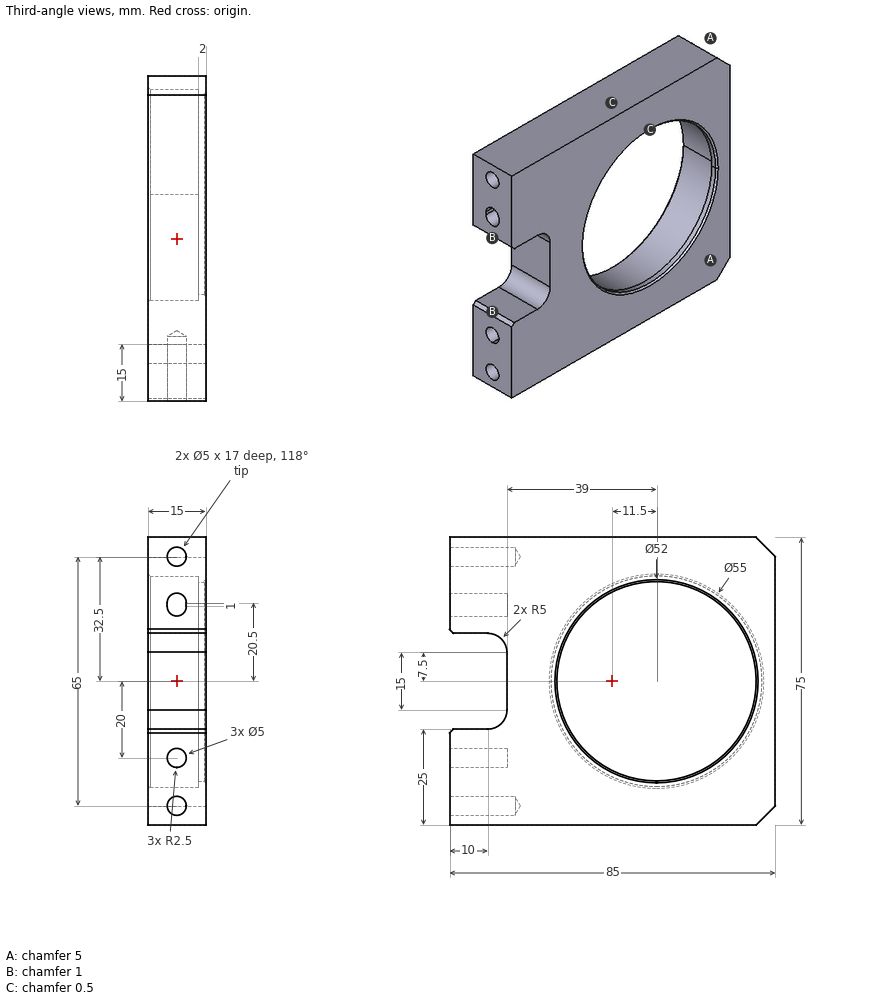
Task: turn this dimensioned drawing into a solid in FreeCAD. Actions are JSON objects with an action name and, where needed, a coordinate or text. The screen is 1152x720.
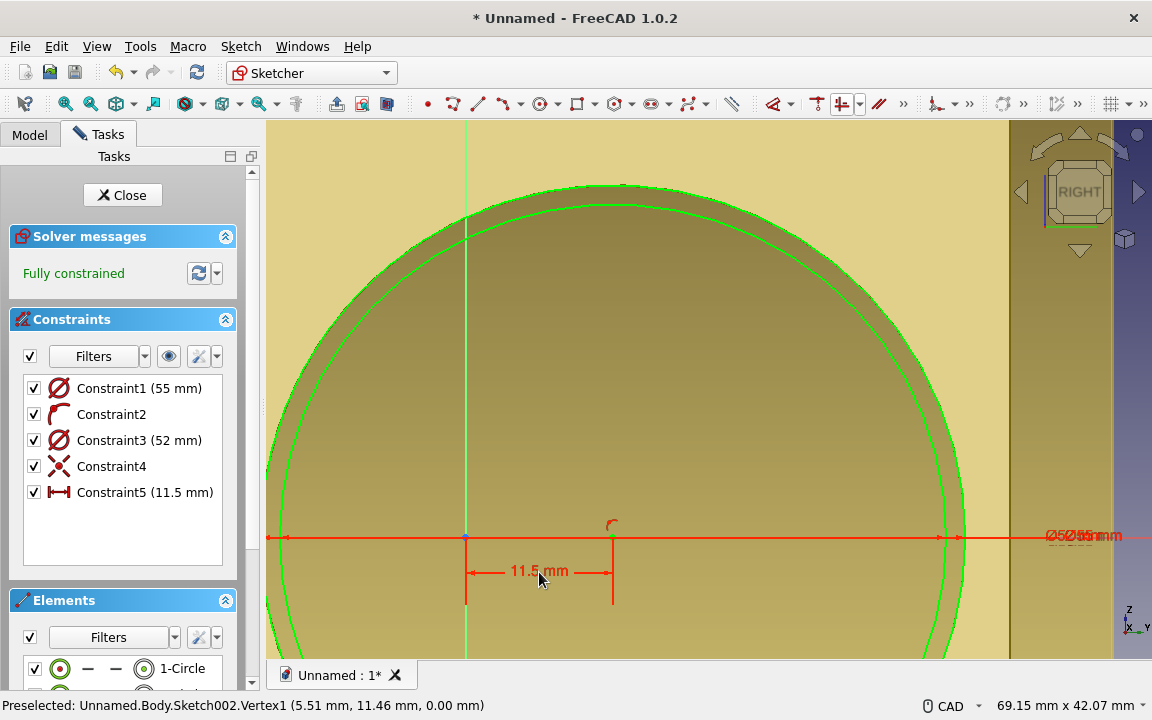
{"action": "left_click", "coordinate": [123, 195]}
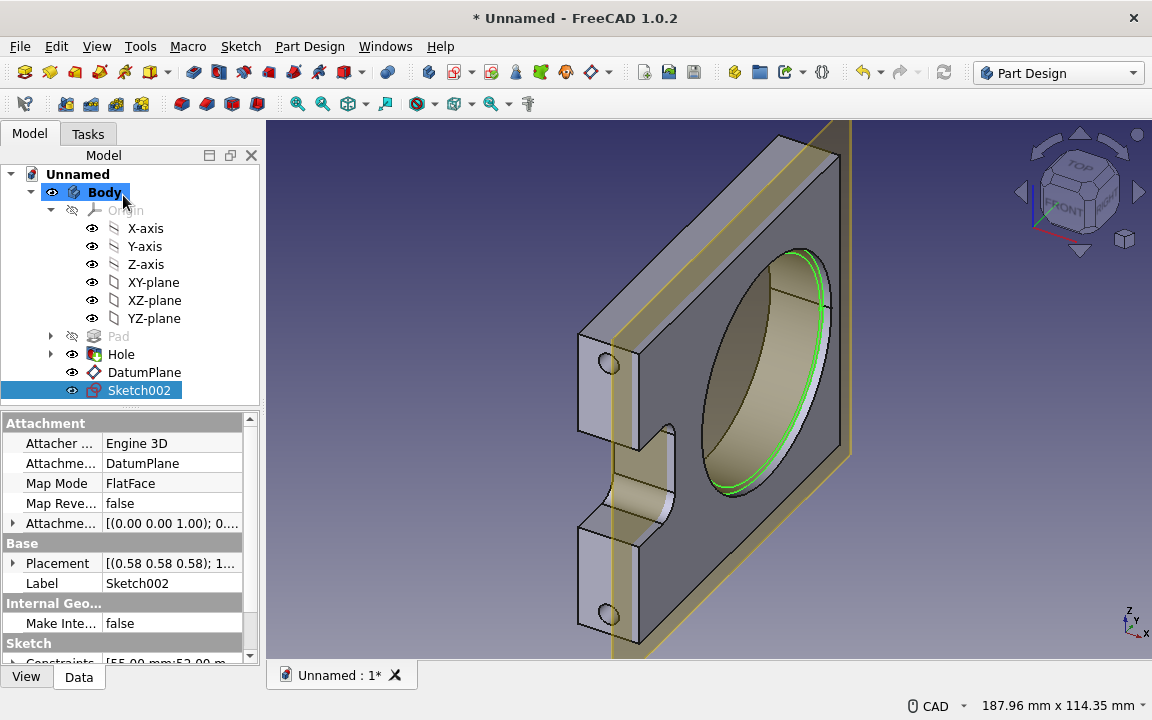
{"action": "left_click", "coordinate": [25, 72]}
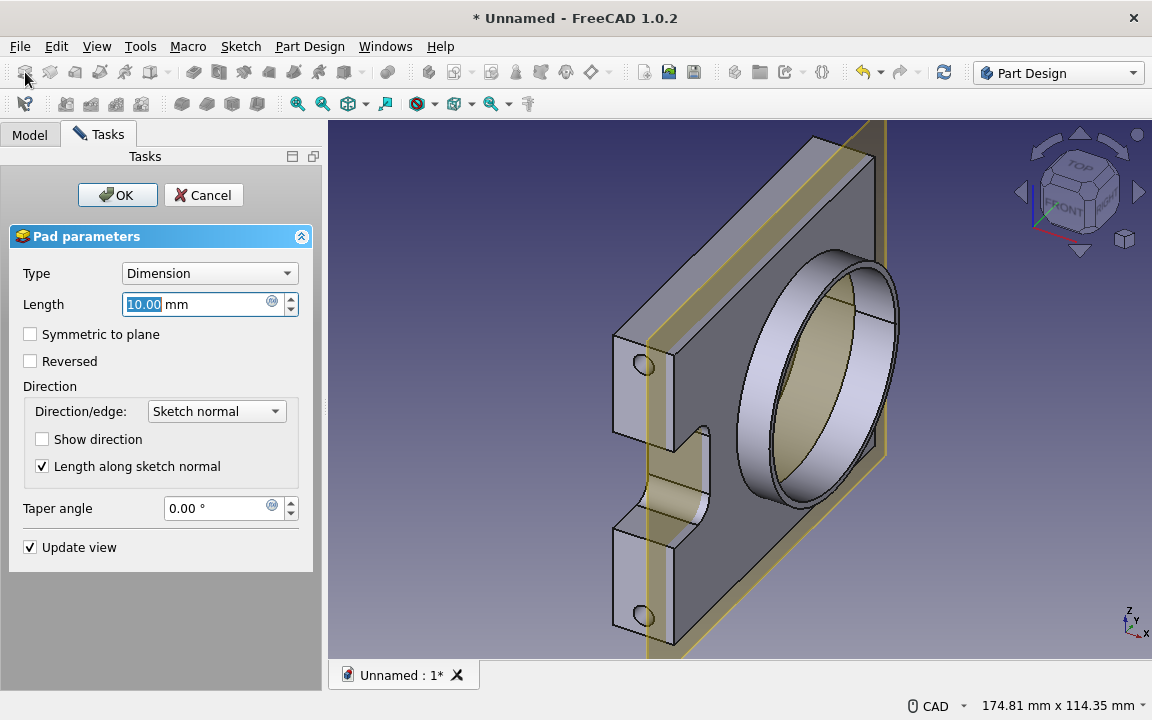
{"action": "type", "text": "2"}
{"action": "key", "text": "Tab"}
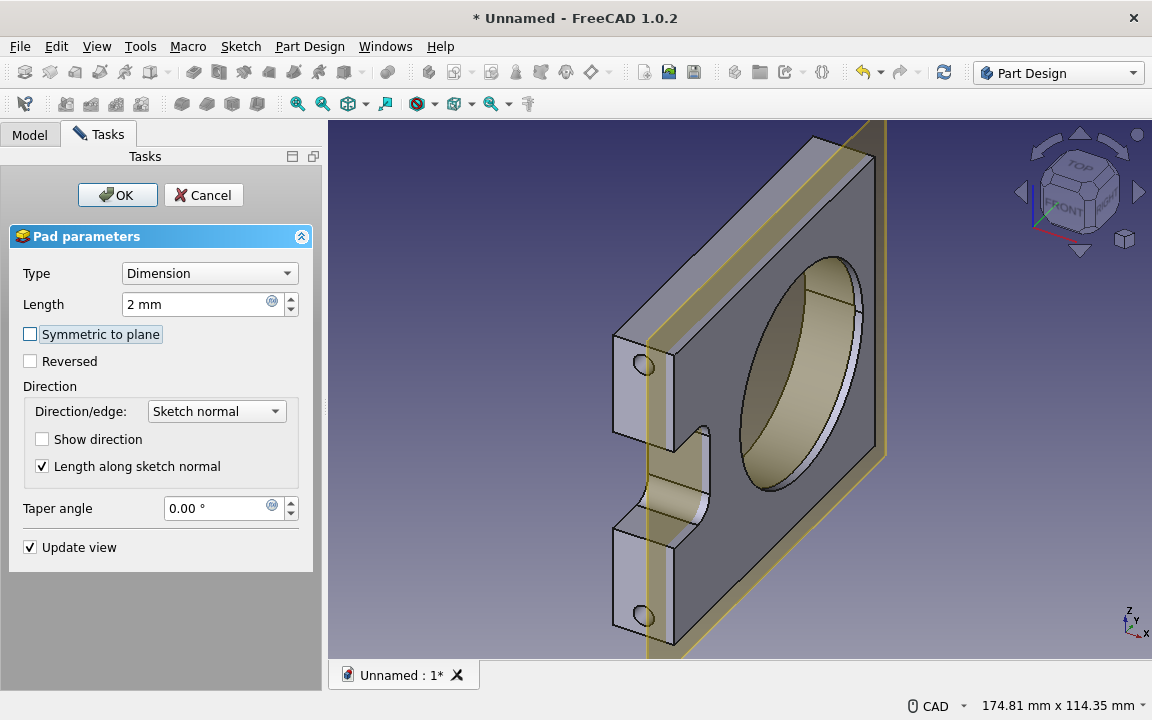
{"action": "left_click", "coordinate": [118, 195]}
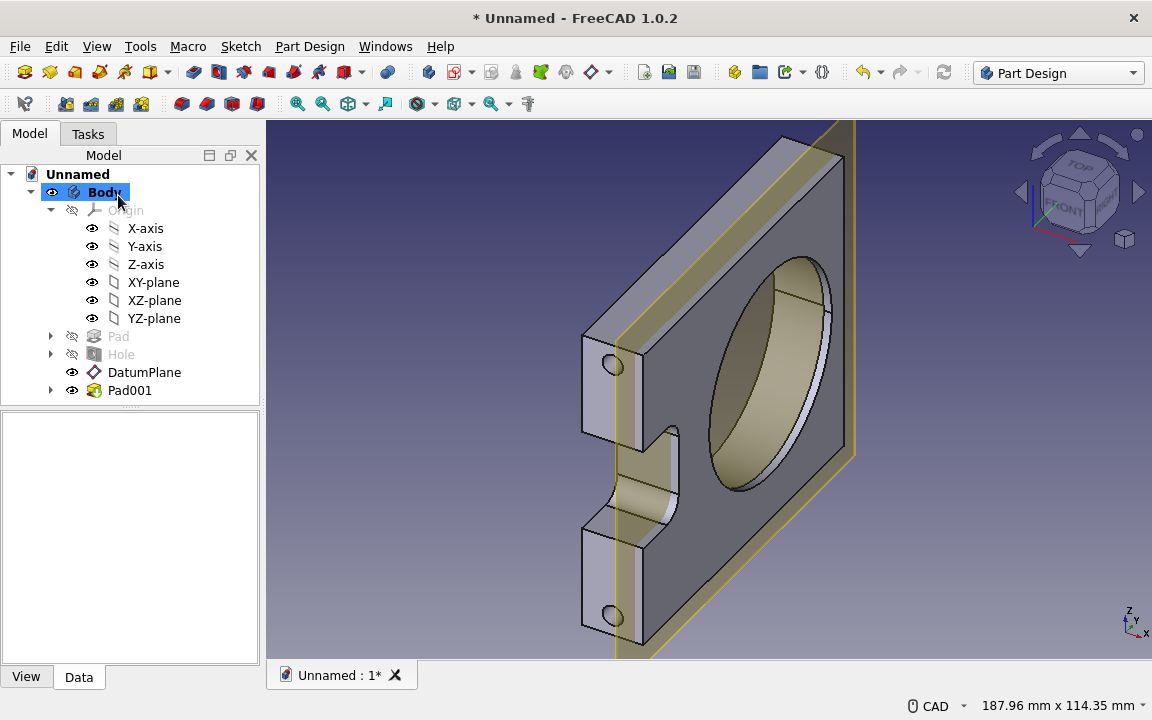
{"action": "left_click", "coordinate": [117, 372]}
{"action": "key", "text": "space"}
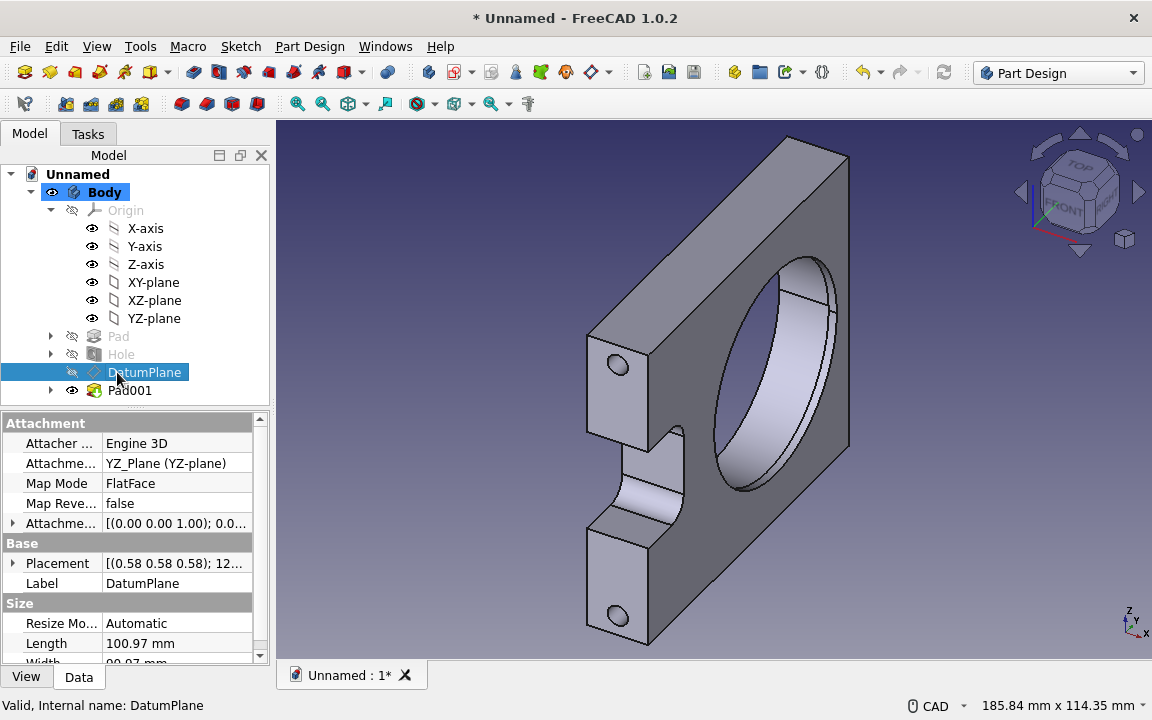
{"action": "key", "text": "0"}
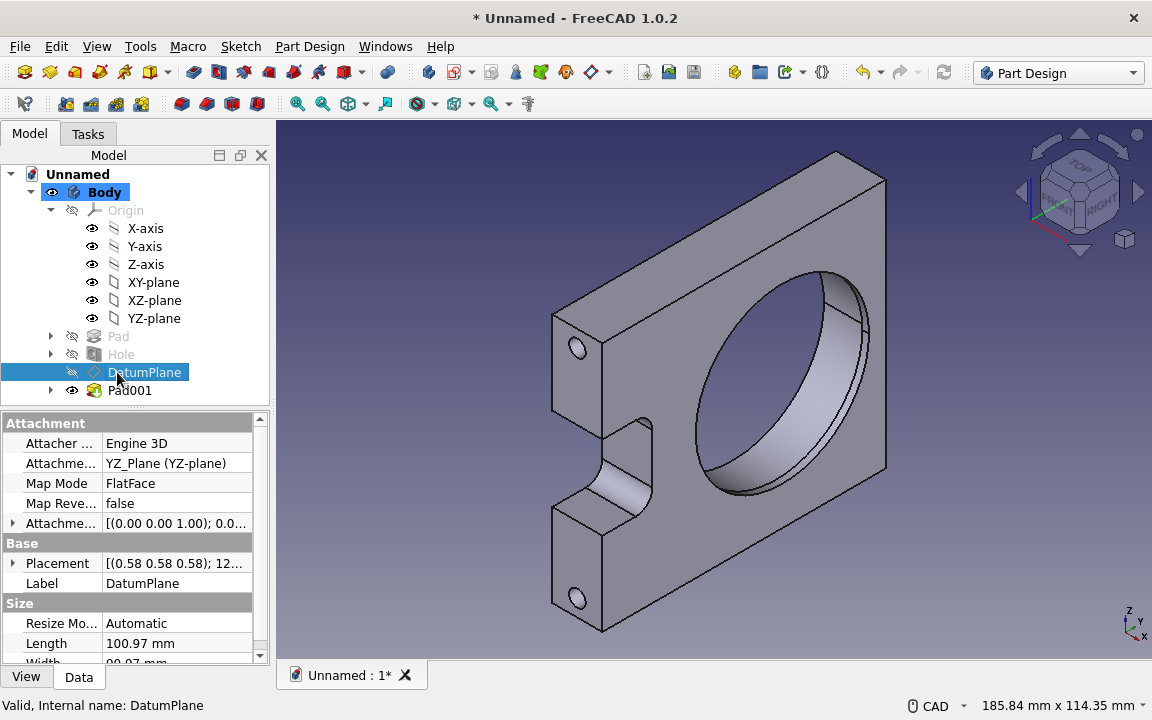
{"action": "key", "text": "2"}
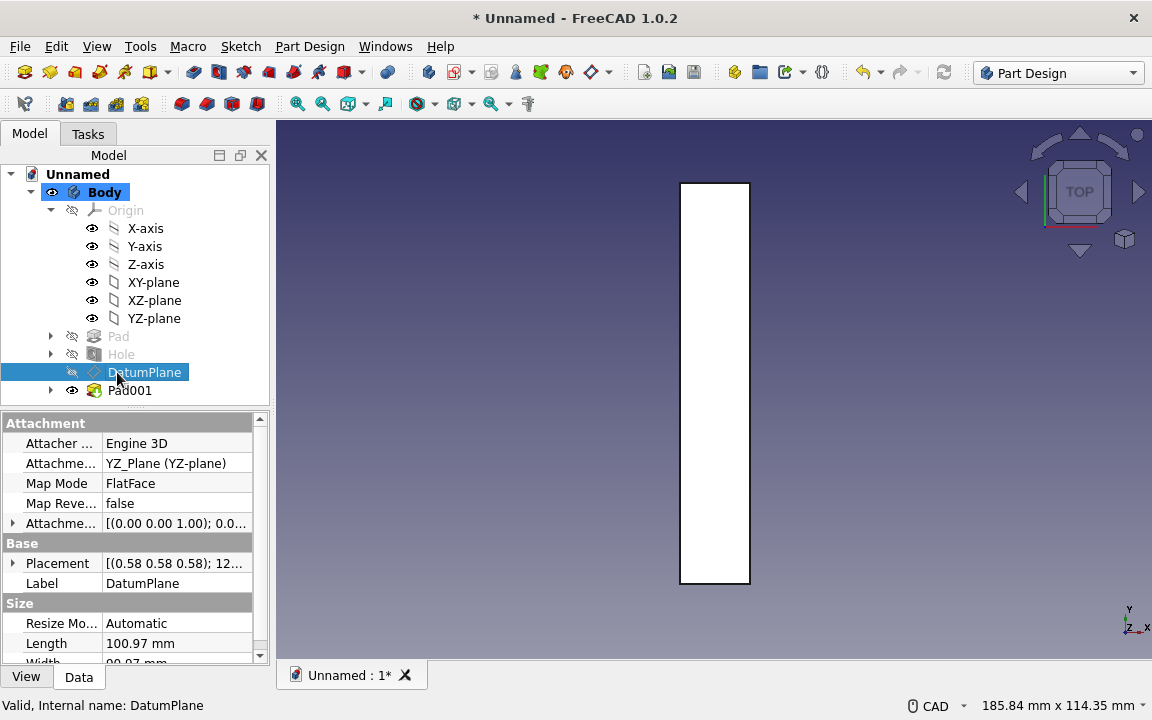
{"action": "left_click", "coordinate": [715, 182]}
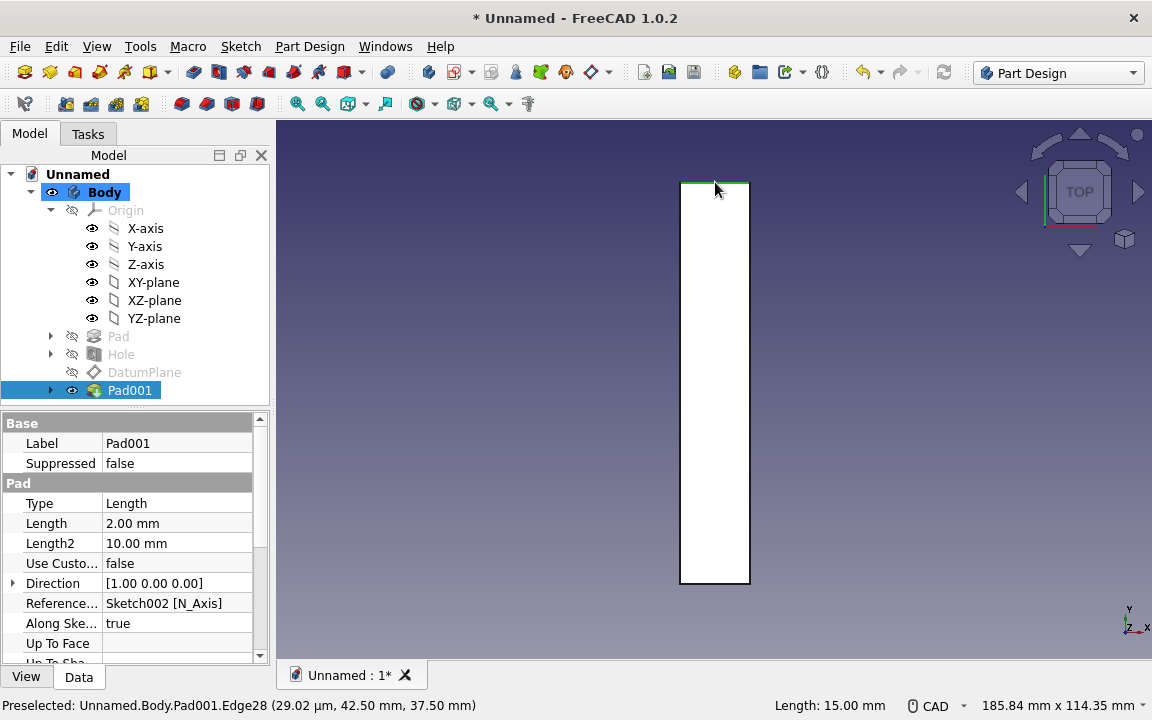
{"action": "key", "text": "1"}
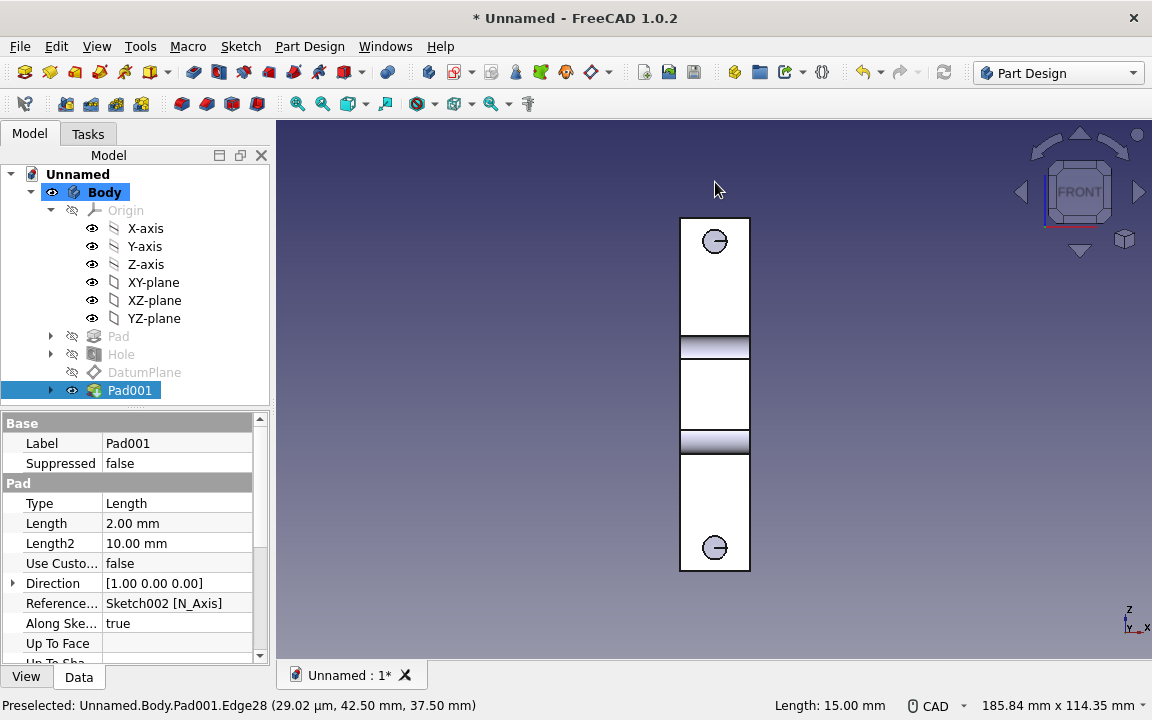
{"action": "key", "text": "3"}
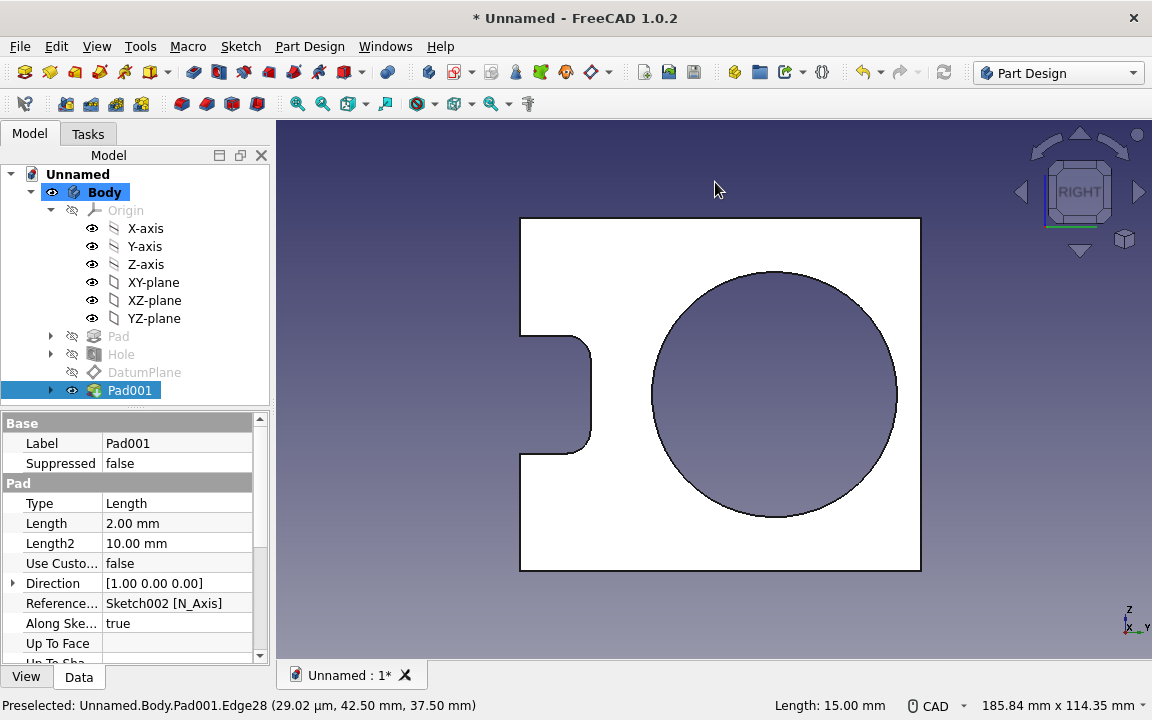
{"action": "key", "text": "5"}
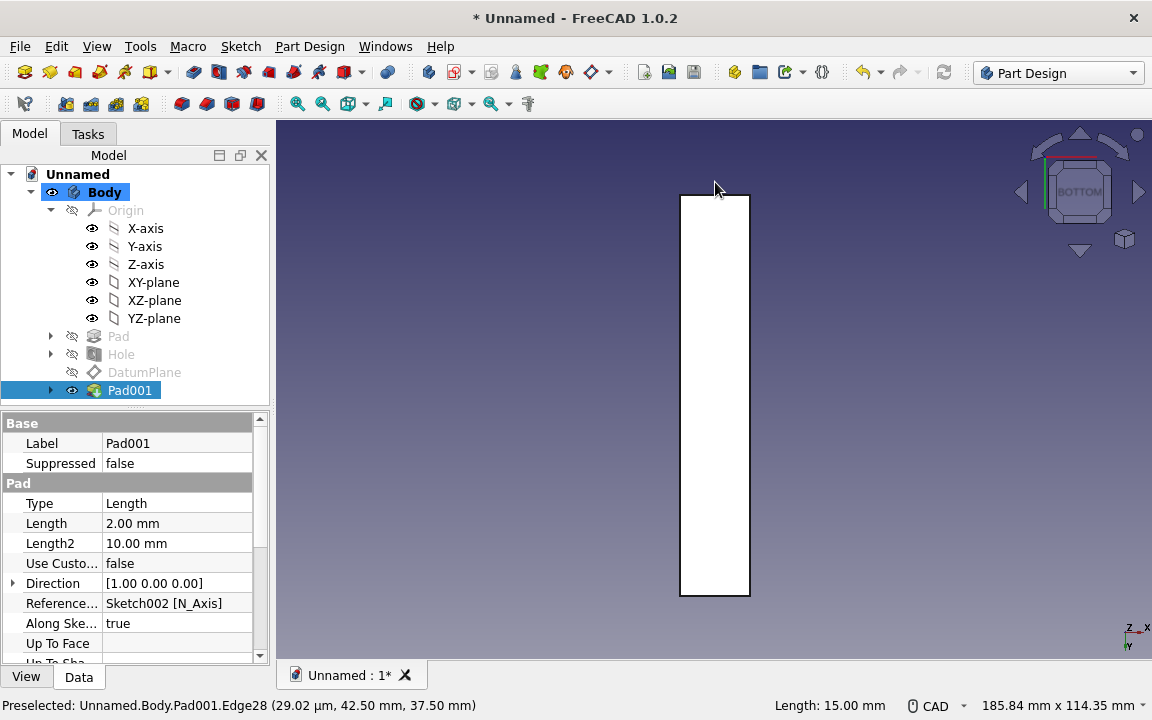
{"action": "left_click", "coordinate": [715, 595], "text": "ctrl"}